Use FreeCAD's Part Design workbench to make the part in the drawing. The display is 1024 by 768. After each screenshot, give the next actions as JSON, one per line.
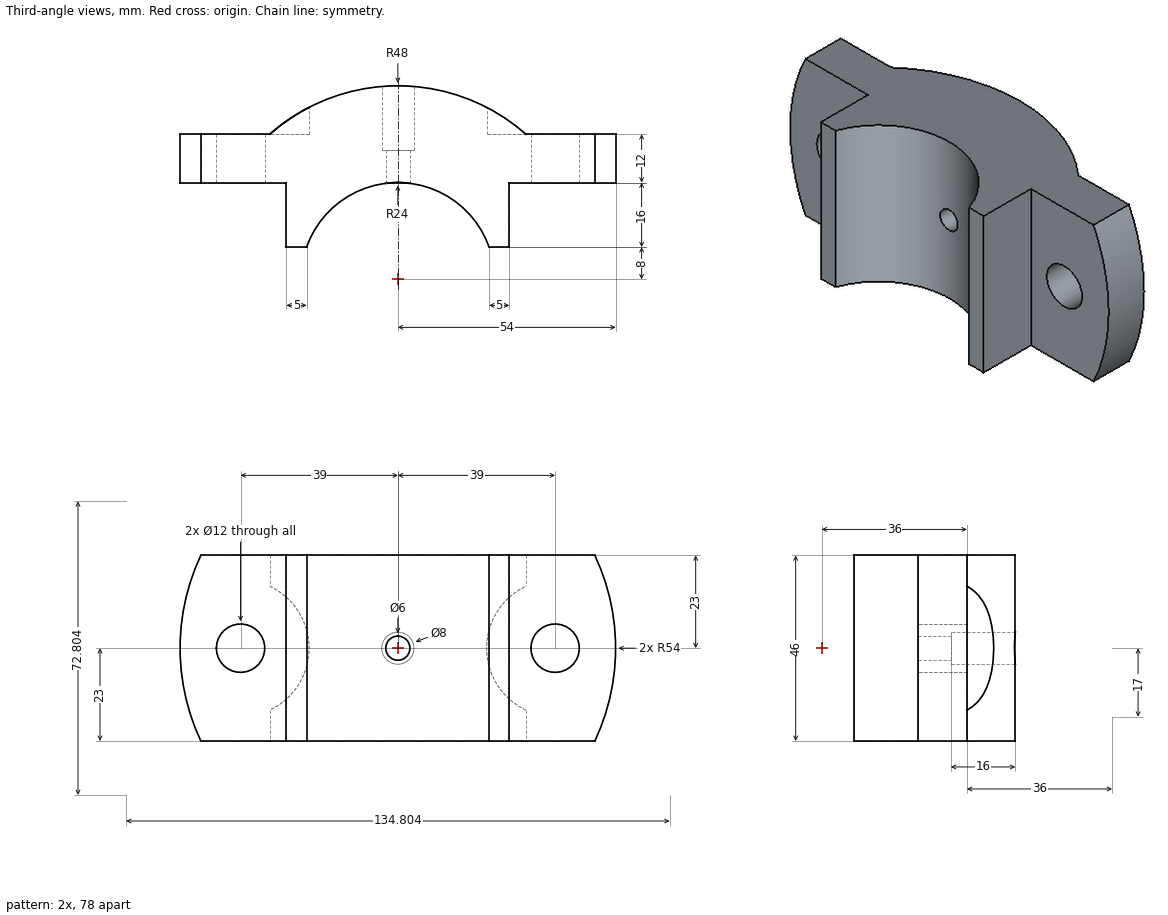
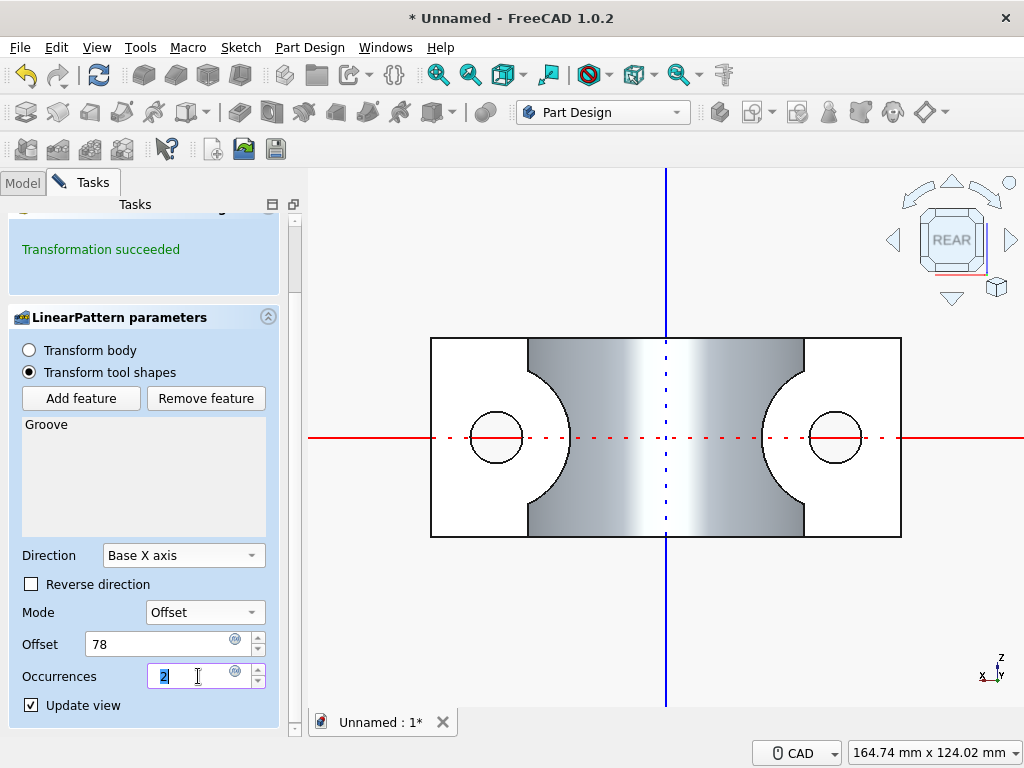
{"action": "type", "text": "2"}
{"action": "key", "text": "Tab"}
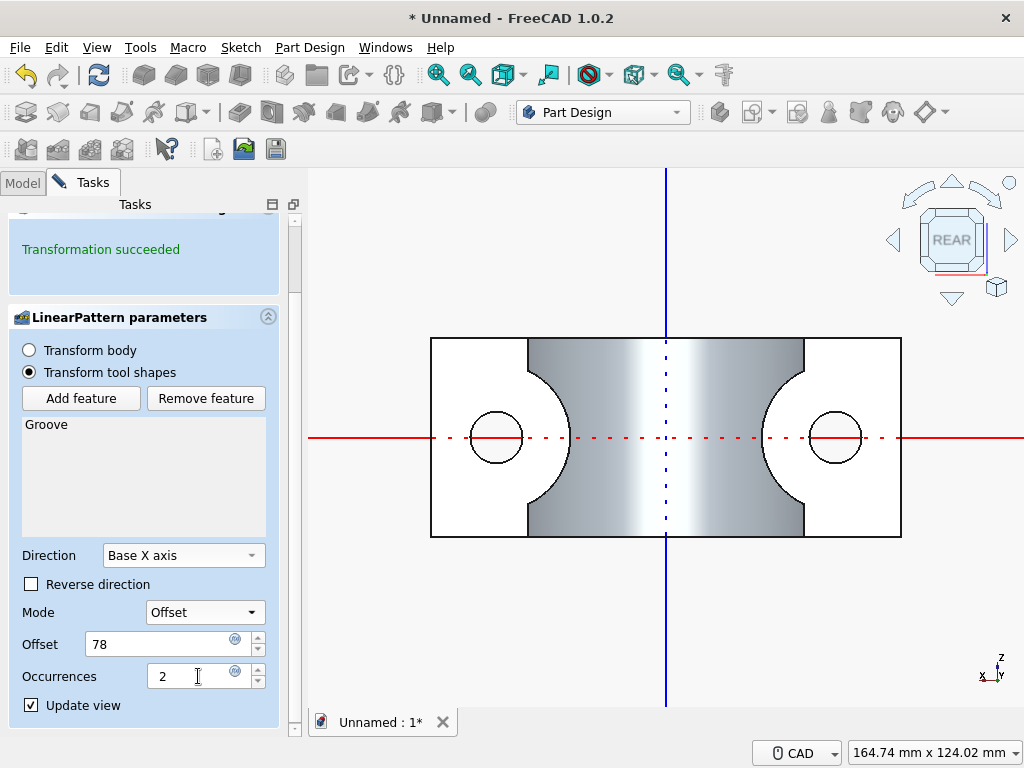
{"action": "scroll", "coordinate": [295, 475], "scroll_direction": "up", "scroll_amount": 3}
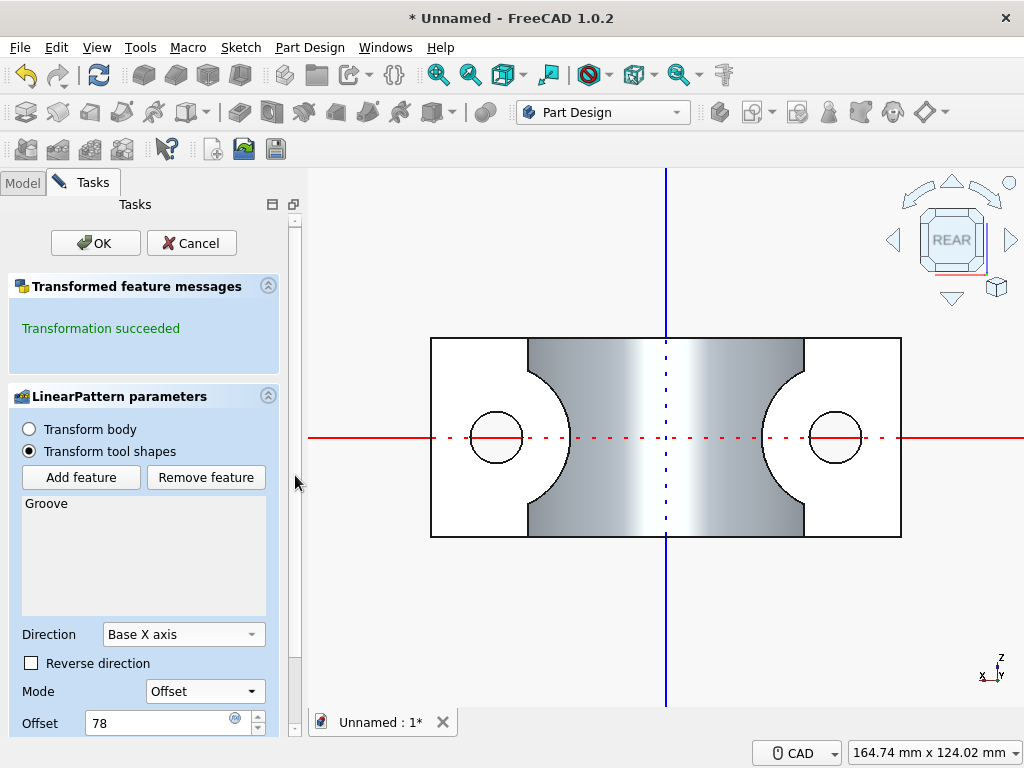
{"action": "left_click", "coordinate": [96, 243]}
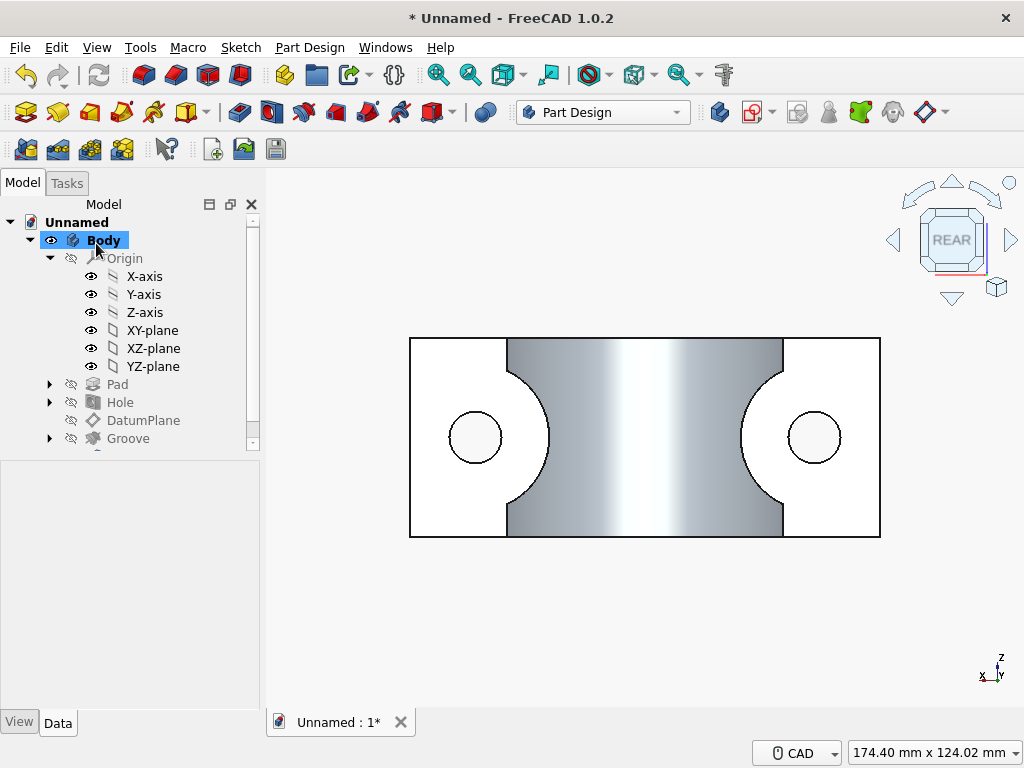
{"action": "left_click", "coordinate": [136, 348]}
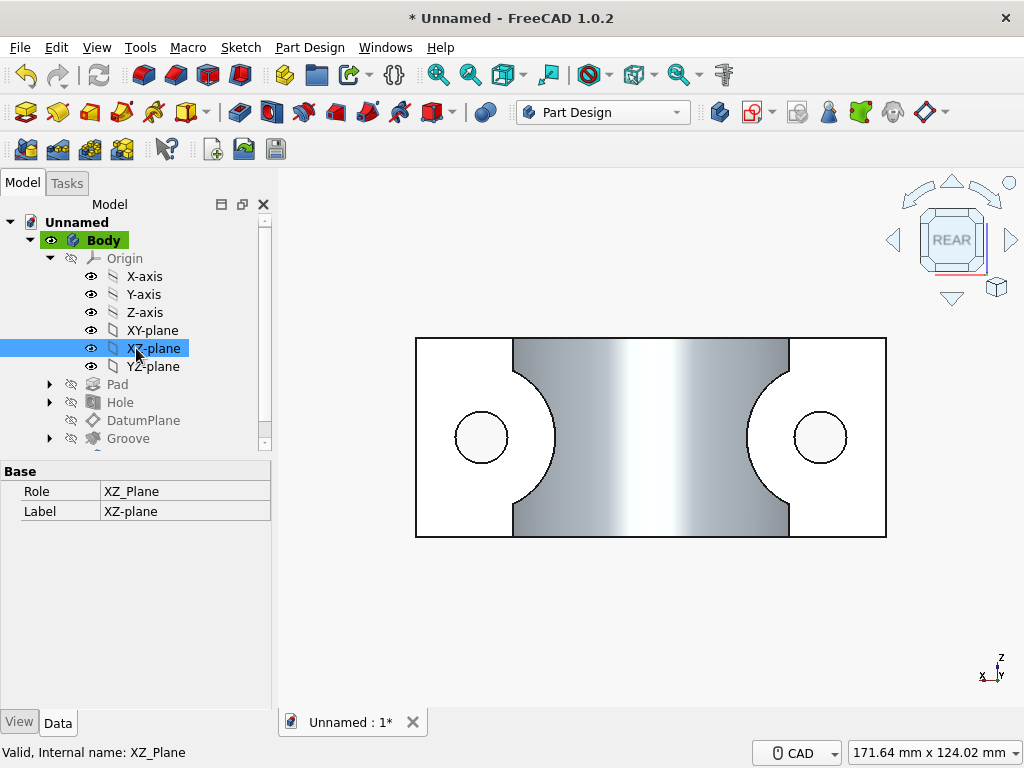
{"action": "left_click", "coordinate": [926, 112]}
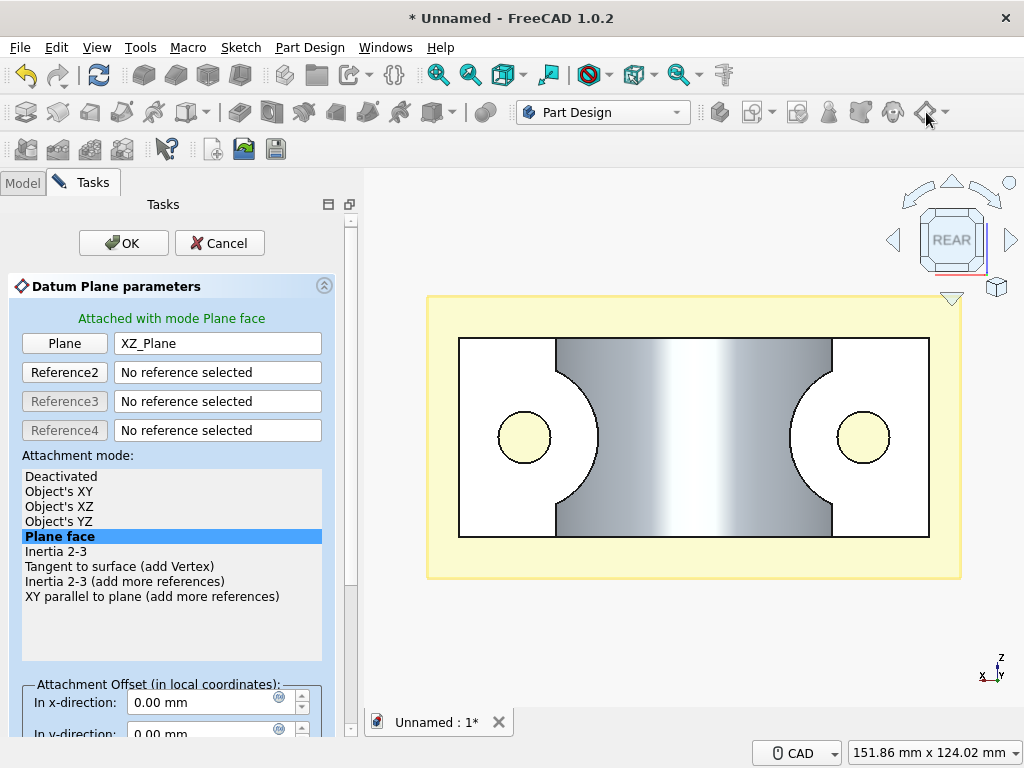
{"action": "scroll", "coordinate": [351, 475], "scroll_direction": "down", "scroll_amount": 2}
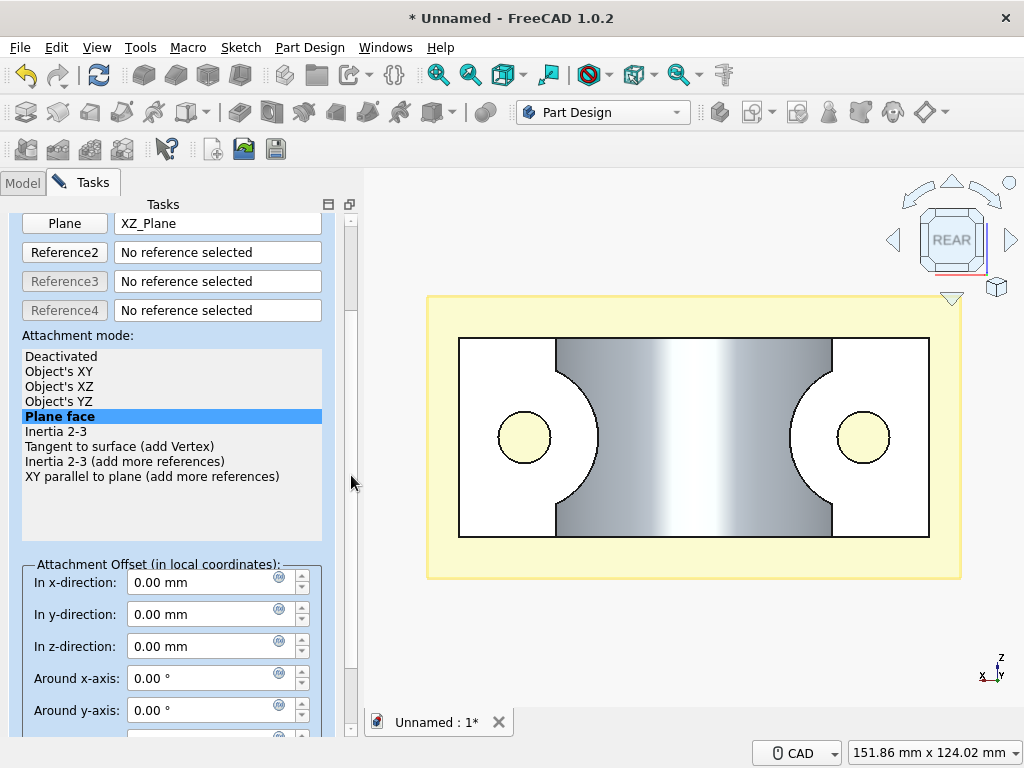
{"action": "triple_click", "coordinate": [210, 646]}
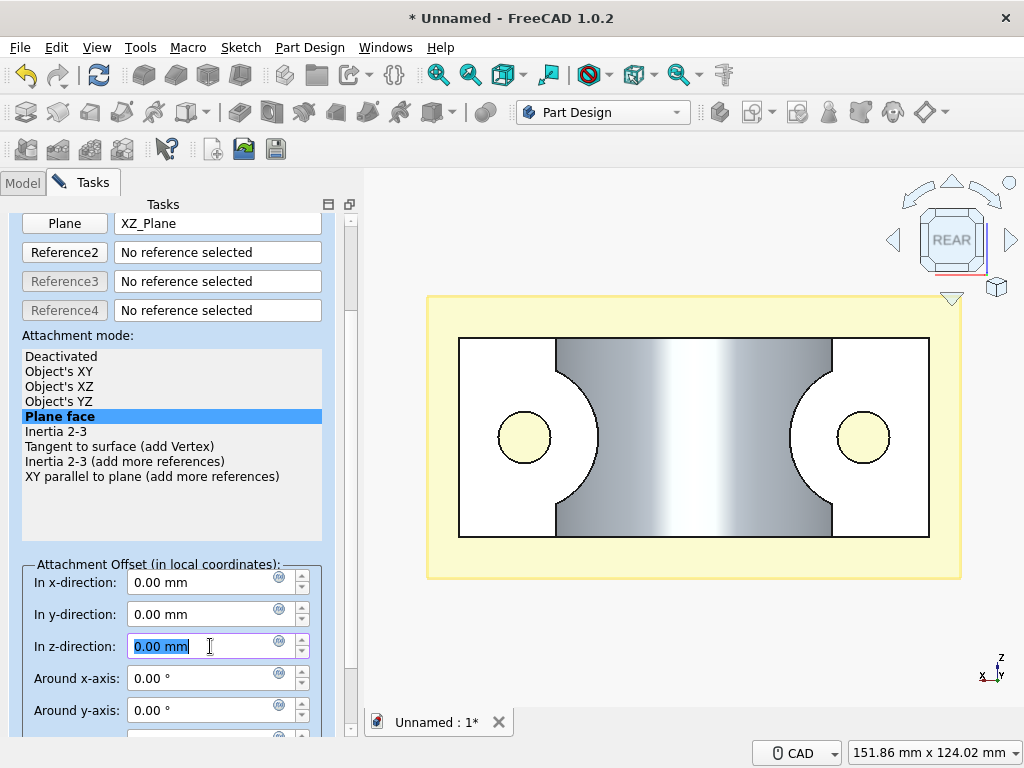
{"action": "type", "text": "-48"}
{"action": "key", "text": "Tab"}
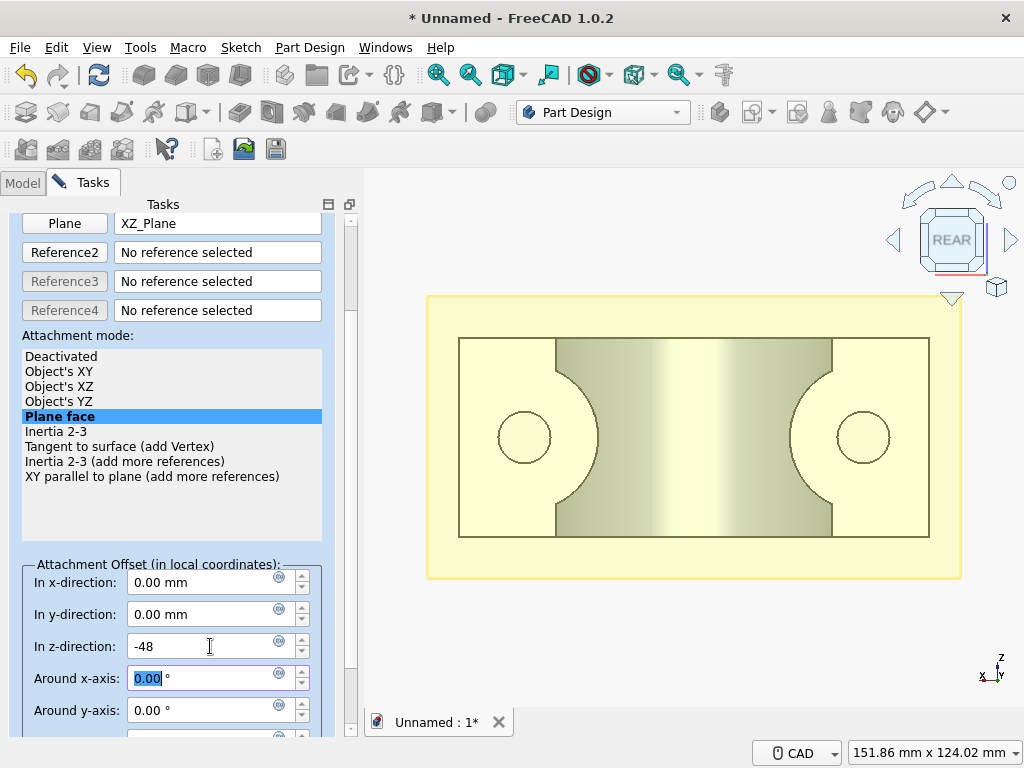
{"action": "scroll", "coordinate": [351, 475], "scroll_direction": "up", "scroll_amount": 3}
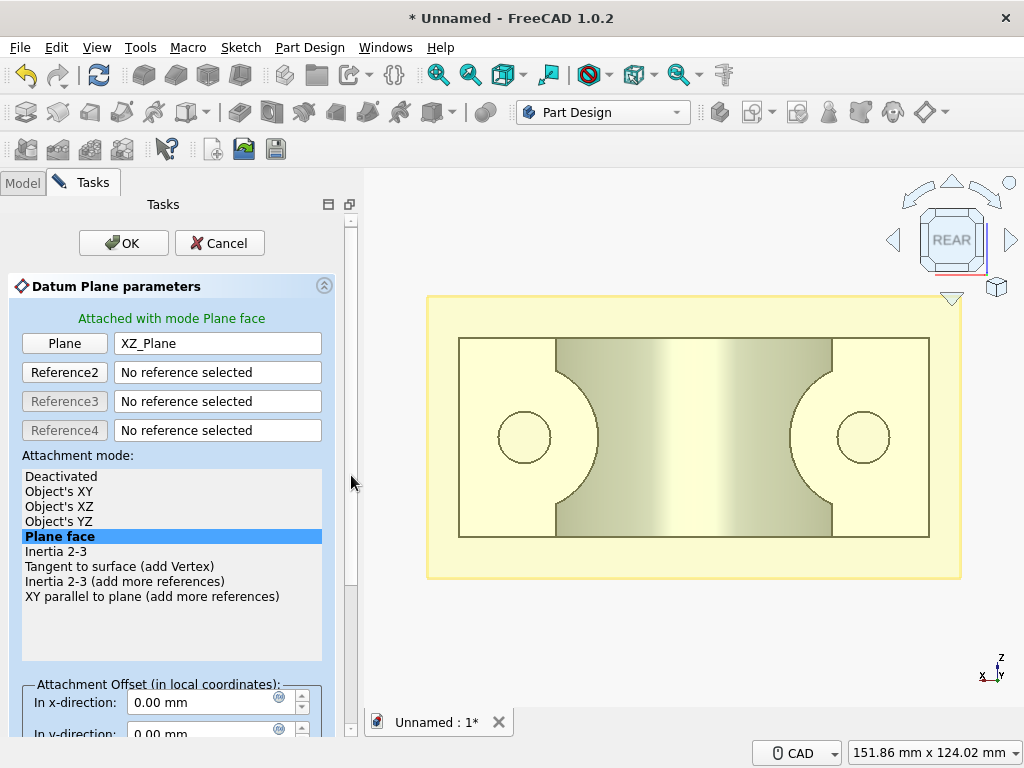
{"action": "left_click", "coordinate": [124, 243]}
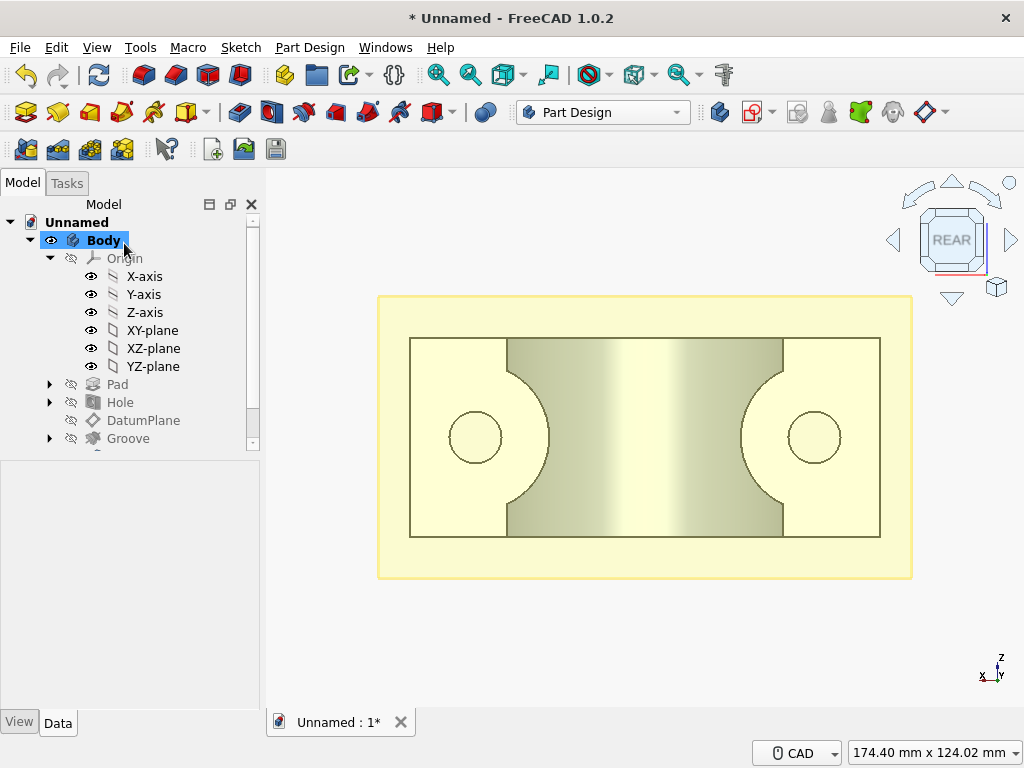
{"action": "scroll", "coordinate": [100, 326], "scroll_direction": "down", "scroll_amount": 3}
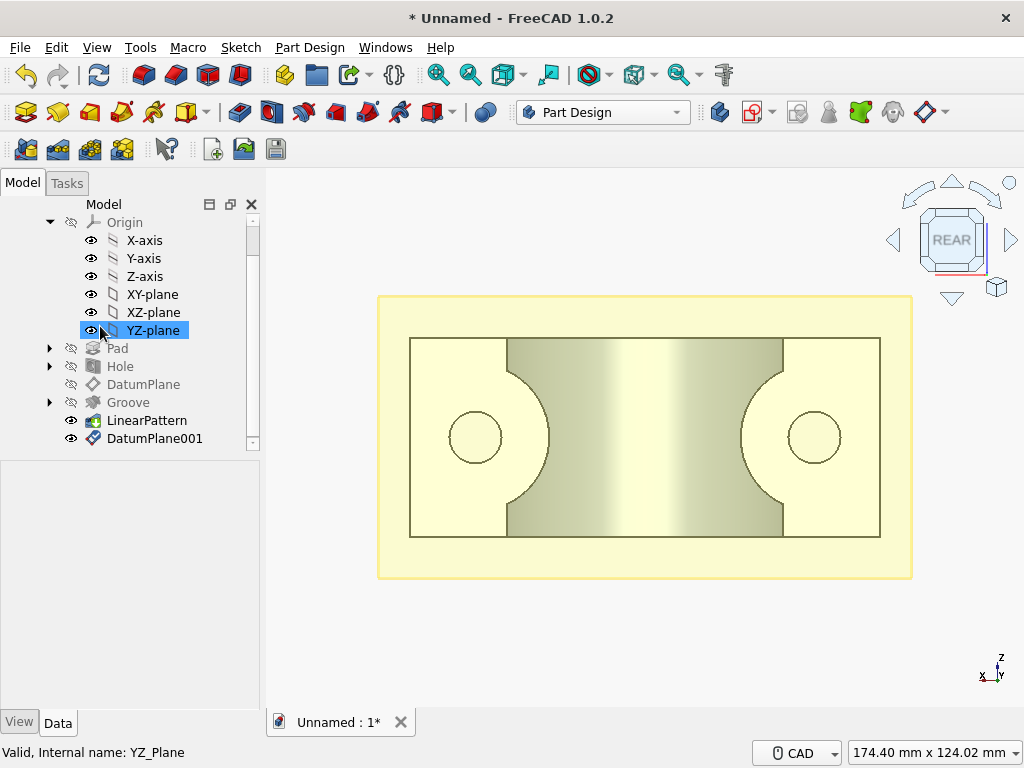
{"action": "left_click", "coordinate": [116, 438]}